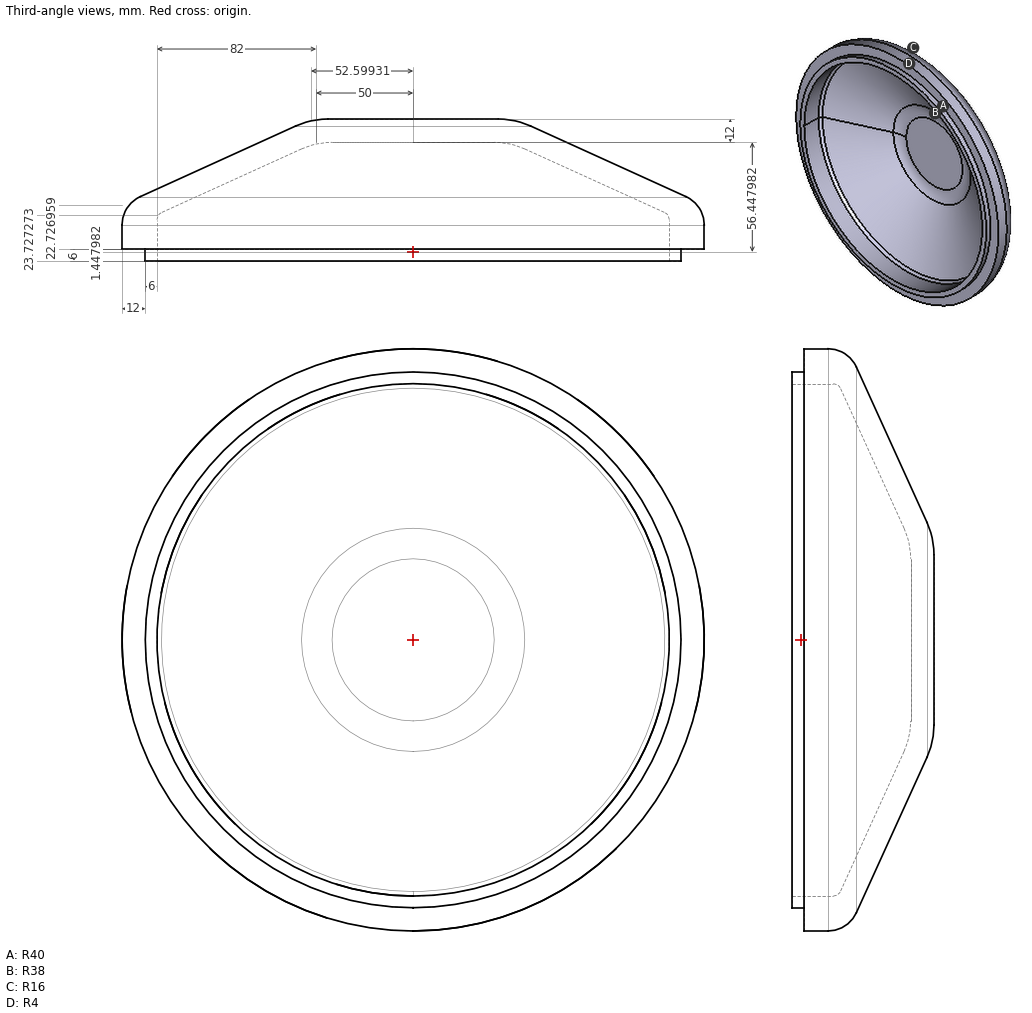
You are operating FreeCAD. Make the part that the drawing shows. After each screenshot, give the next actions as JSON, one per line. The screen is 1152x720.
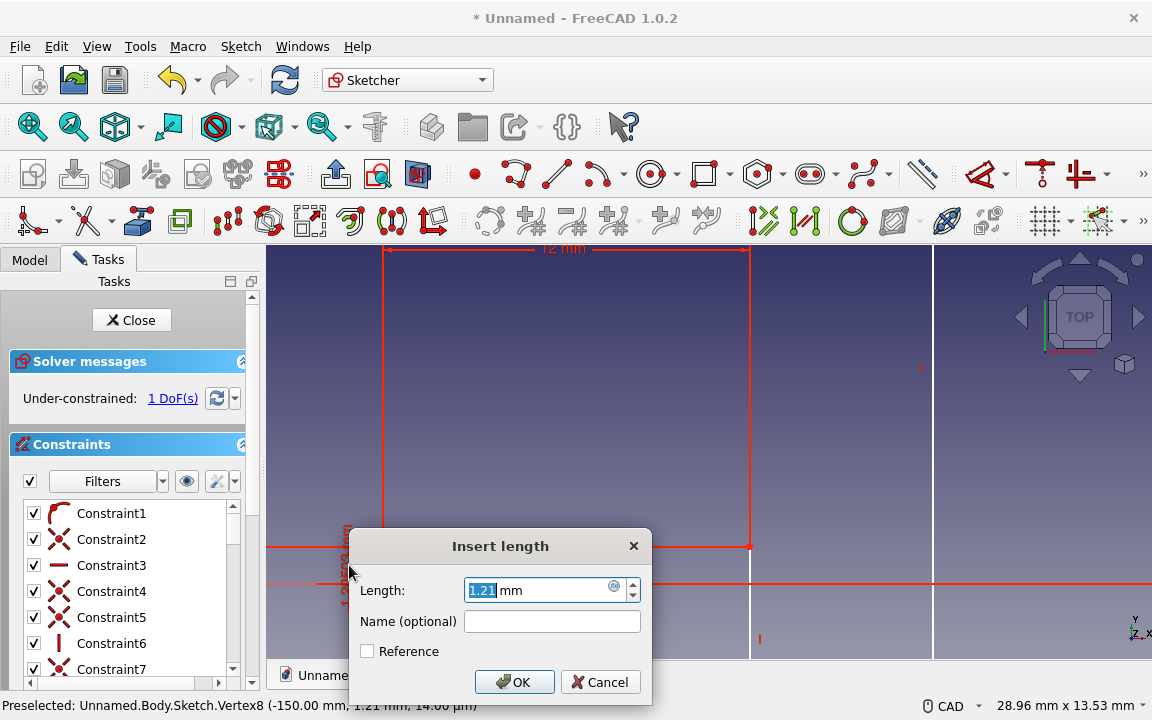
{"action": "type", "text": "1.447982"}
{"action": "key", "text": "Return"}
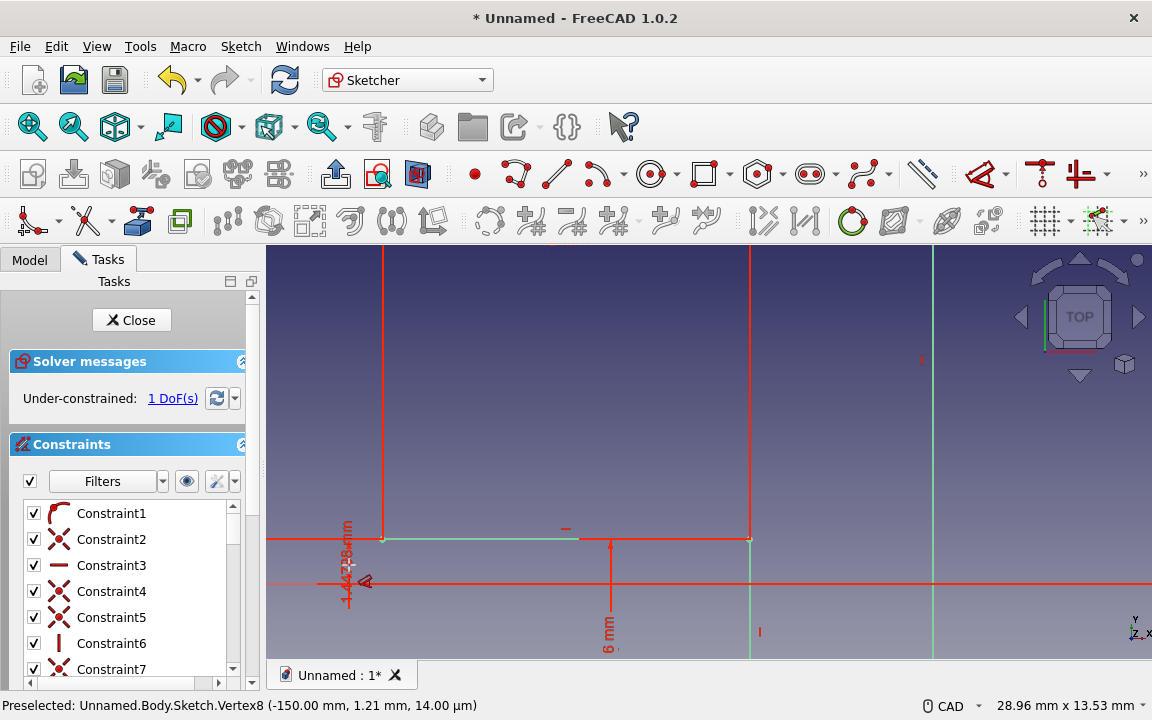
{"action": "scroll", "coordinate": [387, 557], "scroll_direction": "down", "scroll_amount": 11}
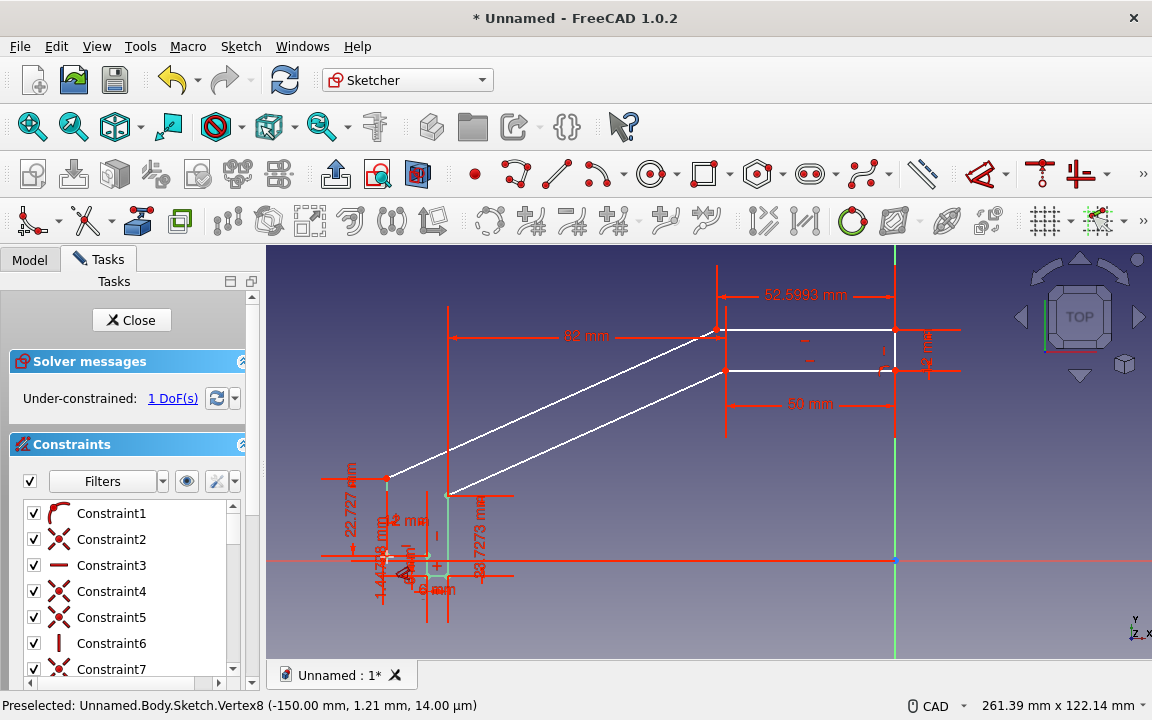
{"action": "left_click", "coordinate": [895, 371]}
{"action": "left_click", "coordinate": [929, 466]}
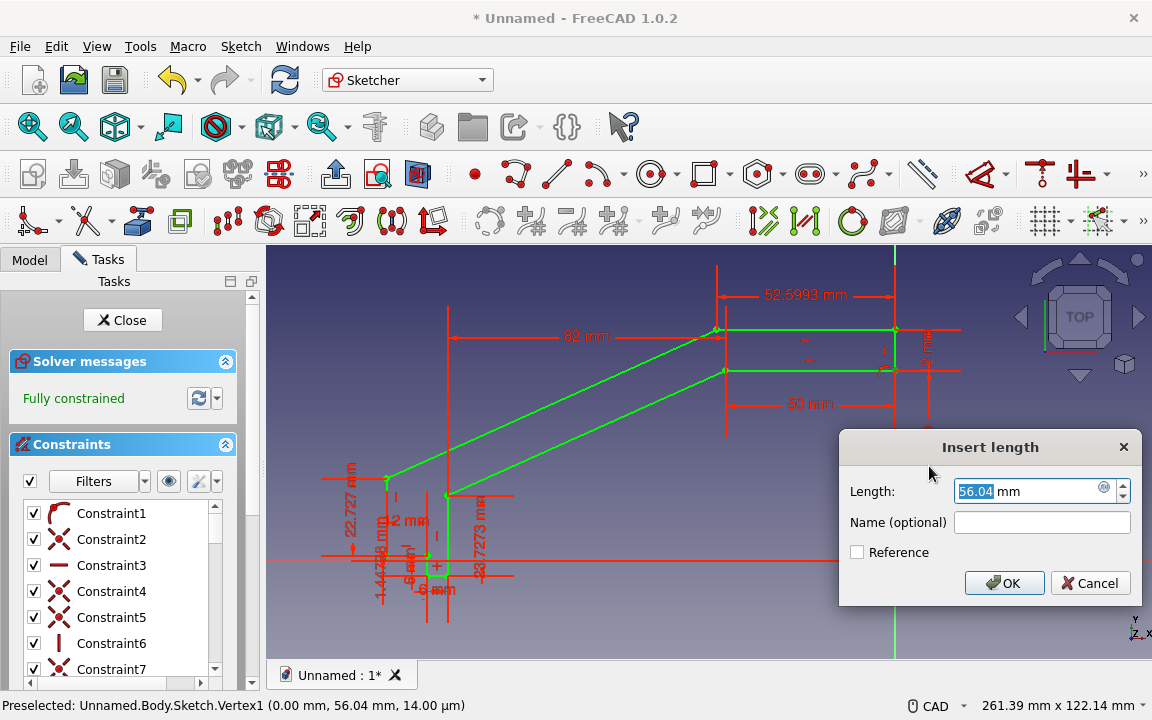
{"action": "type", "text": "56.447982"}
{"action": "key", "text": "Return"}
{"action": "key", "text": "Escape"}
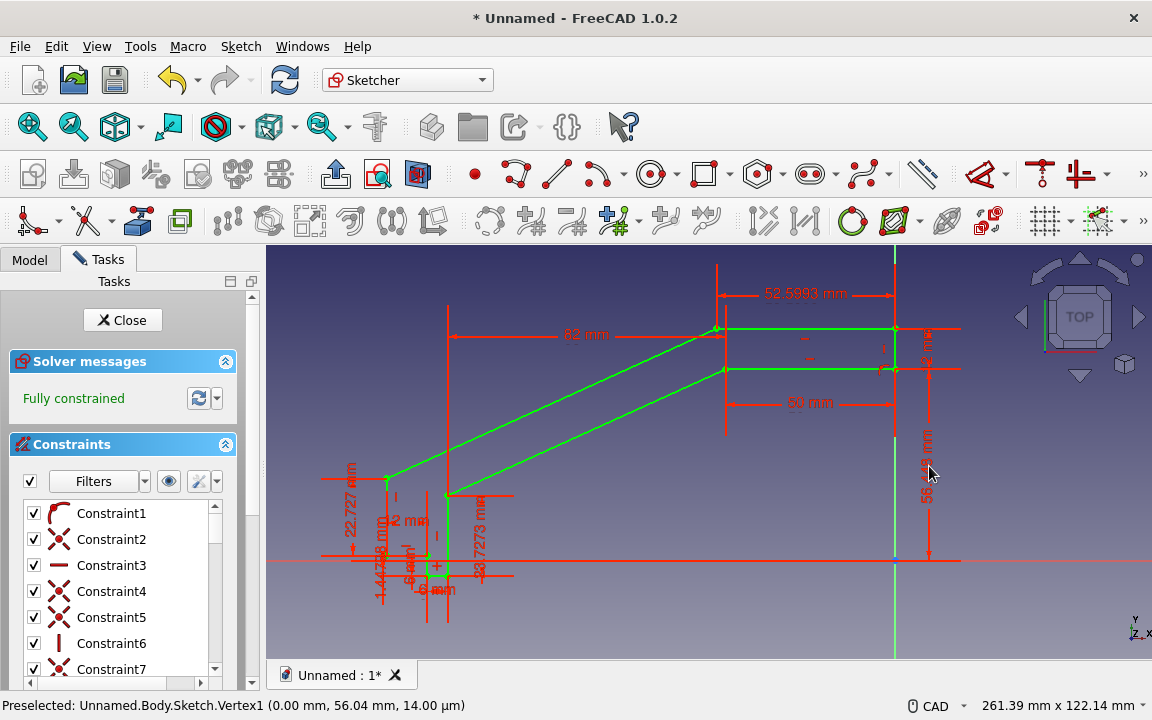
{"action": "left_click", "coordinate": [123, 320]}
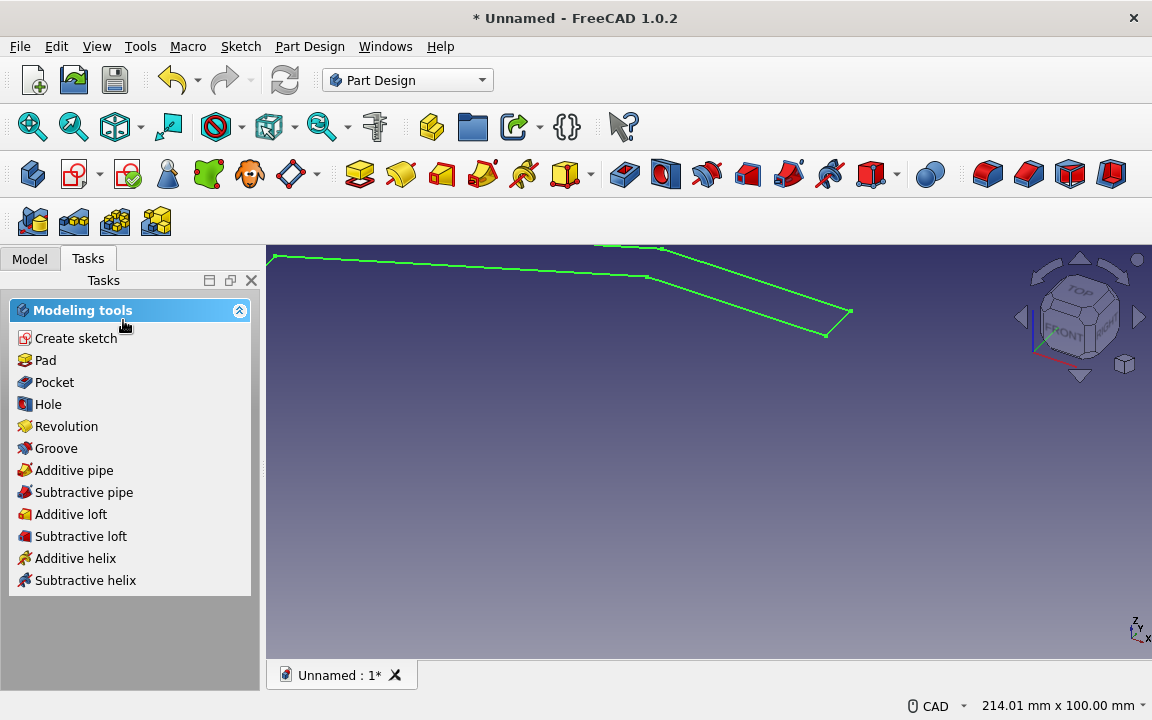
{"action": "left_click", "coordinate": [401, 174]}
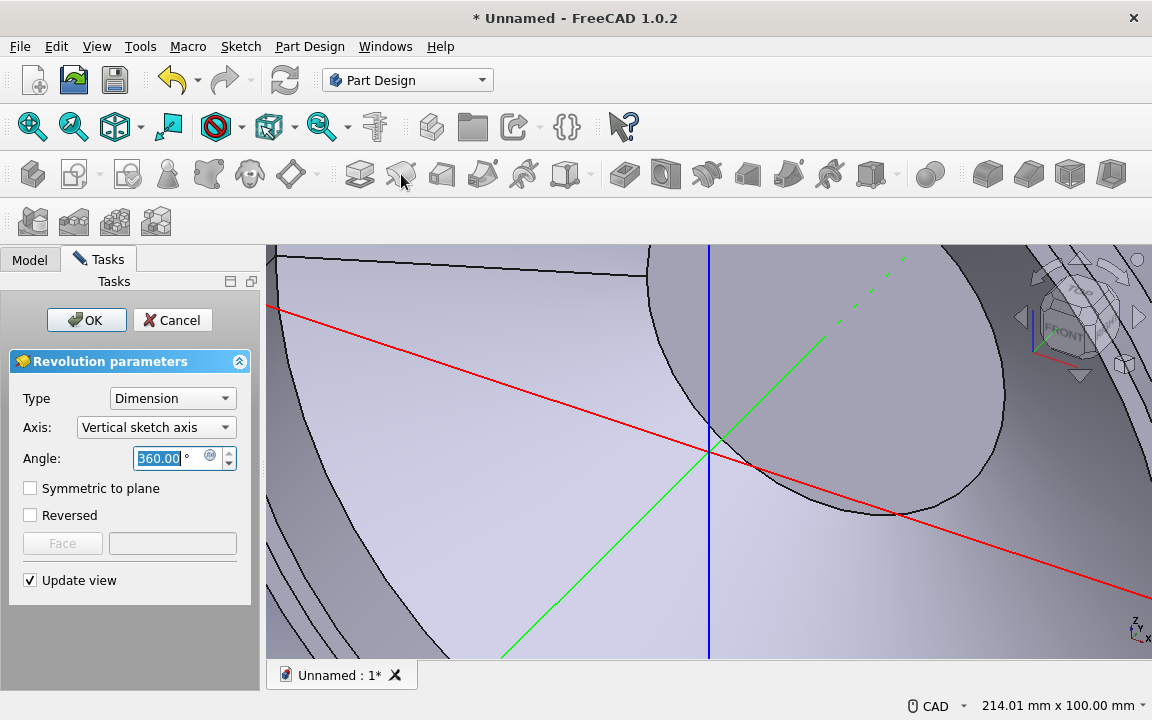
{"action": "left_click", "coordinate": [87, 320]}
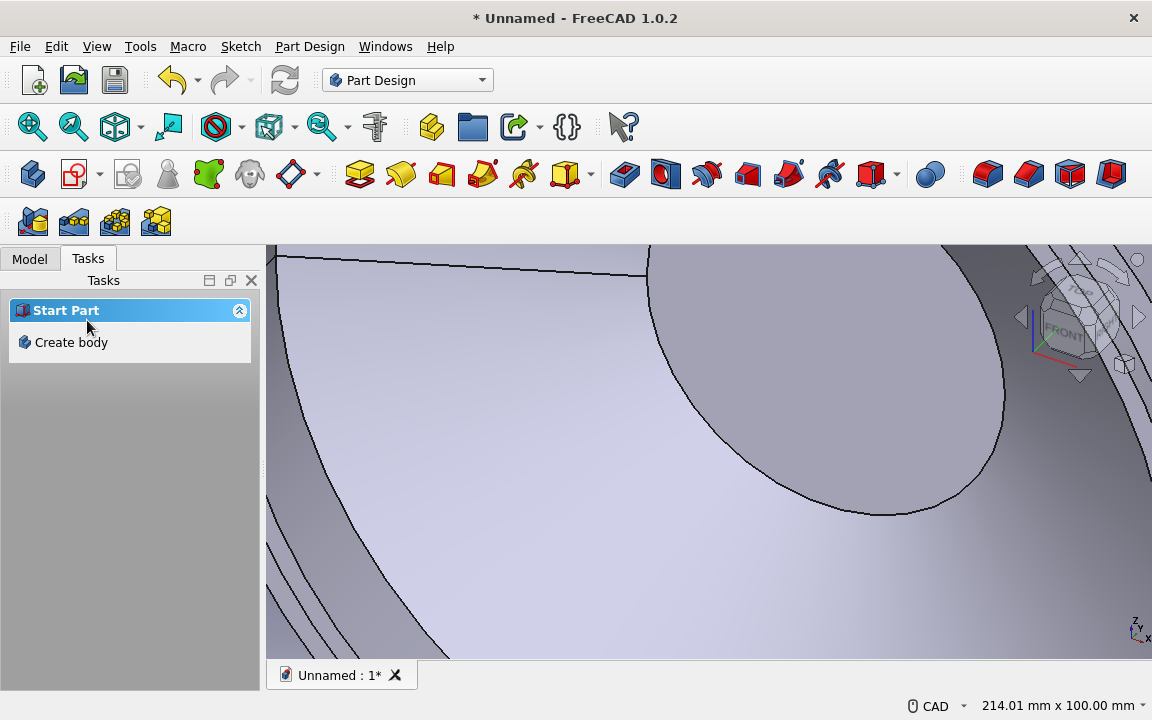
{"action": "left_click", "coordinate": [33, 128]}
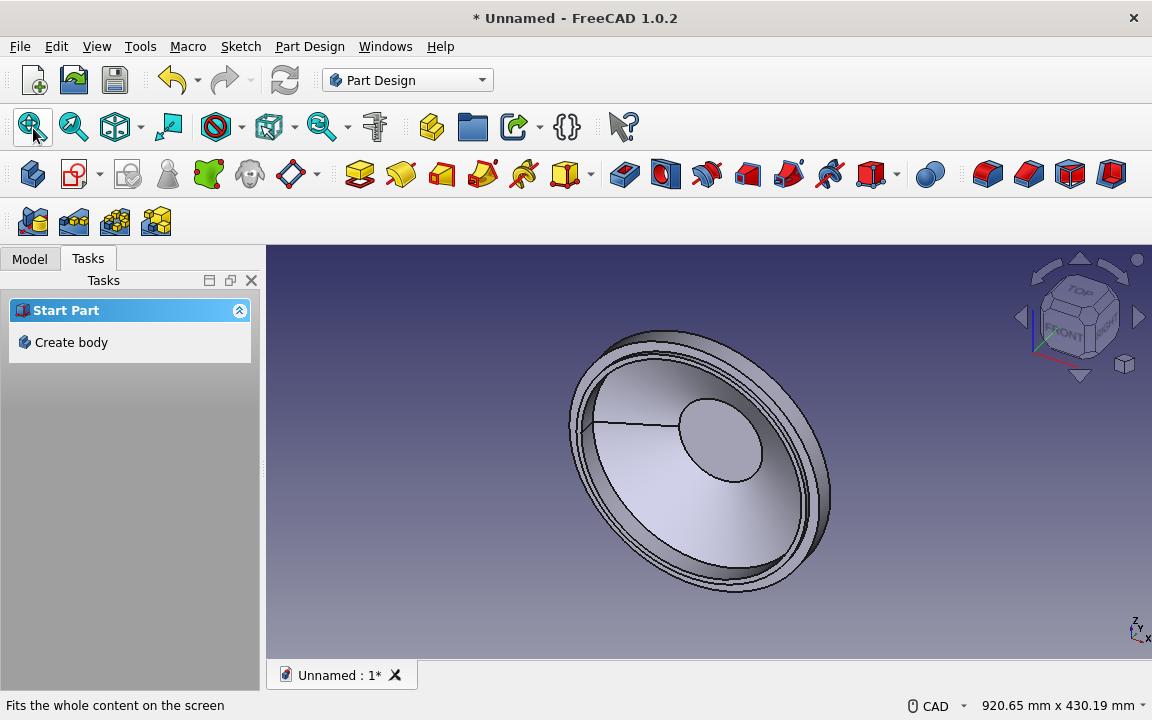
{"action": "key", "text": "0"}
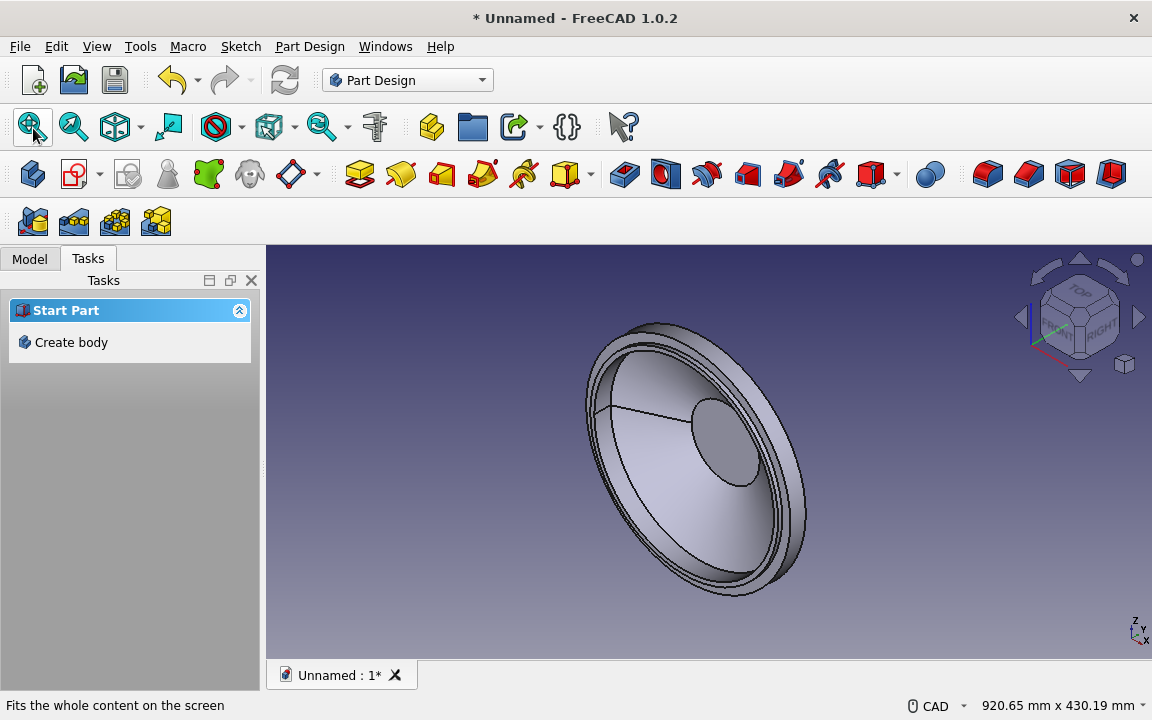
{"action": "key", "text": "2"}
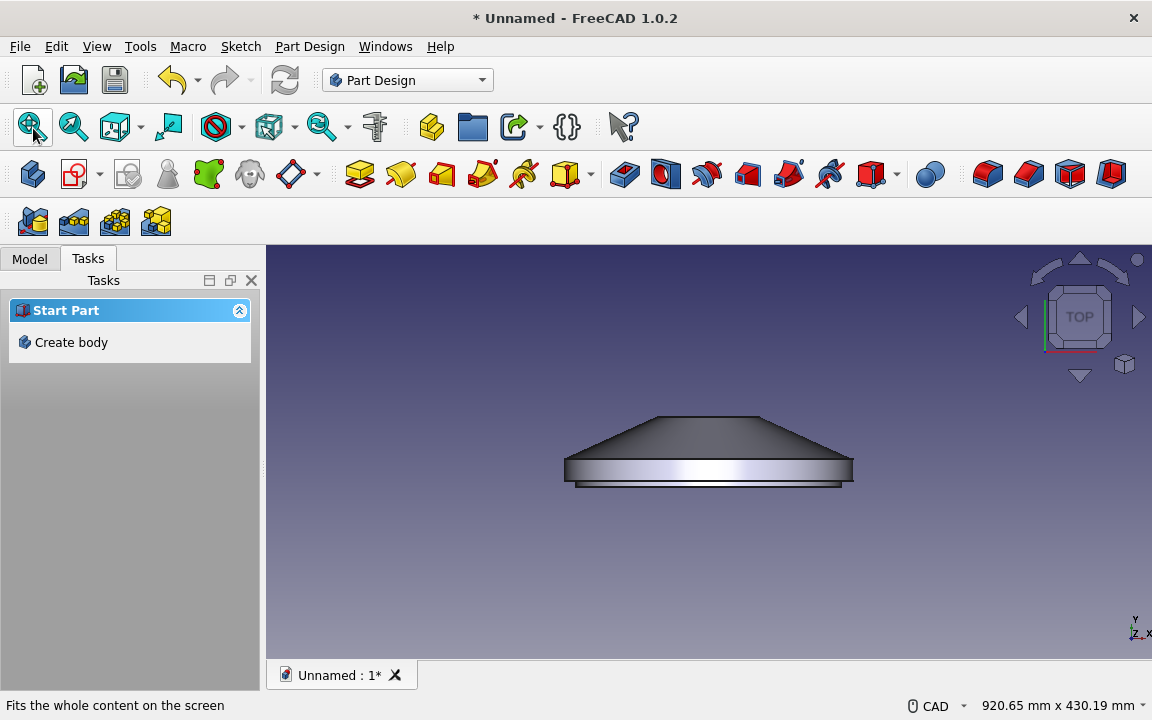
{"action": "key", "text": "v f"}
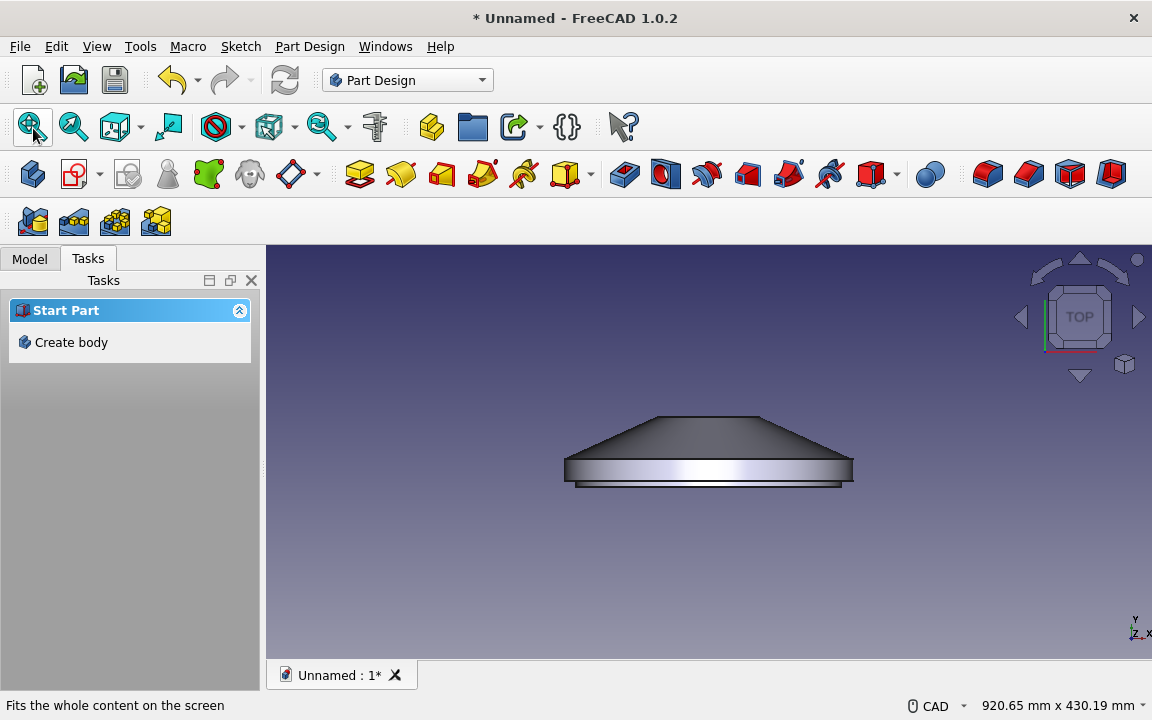
{"action": "key", "text": "1"}